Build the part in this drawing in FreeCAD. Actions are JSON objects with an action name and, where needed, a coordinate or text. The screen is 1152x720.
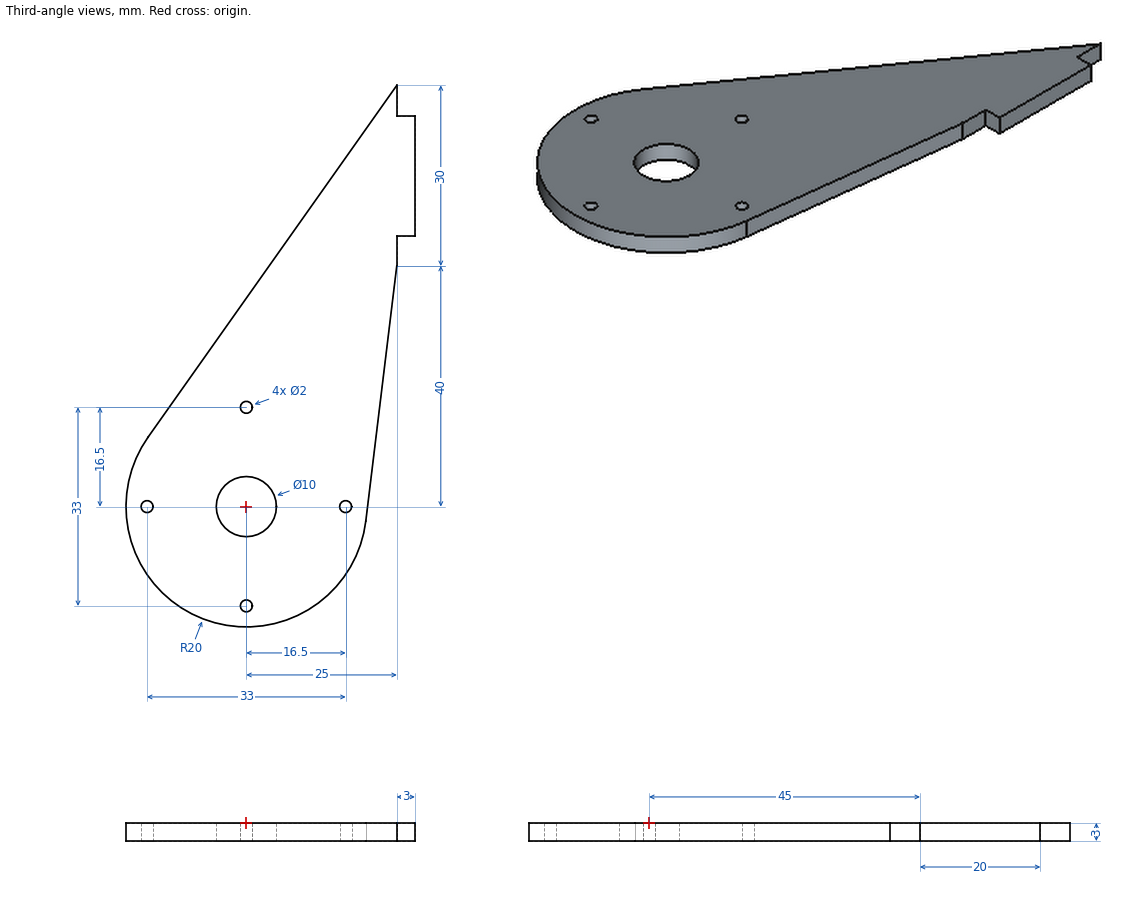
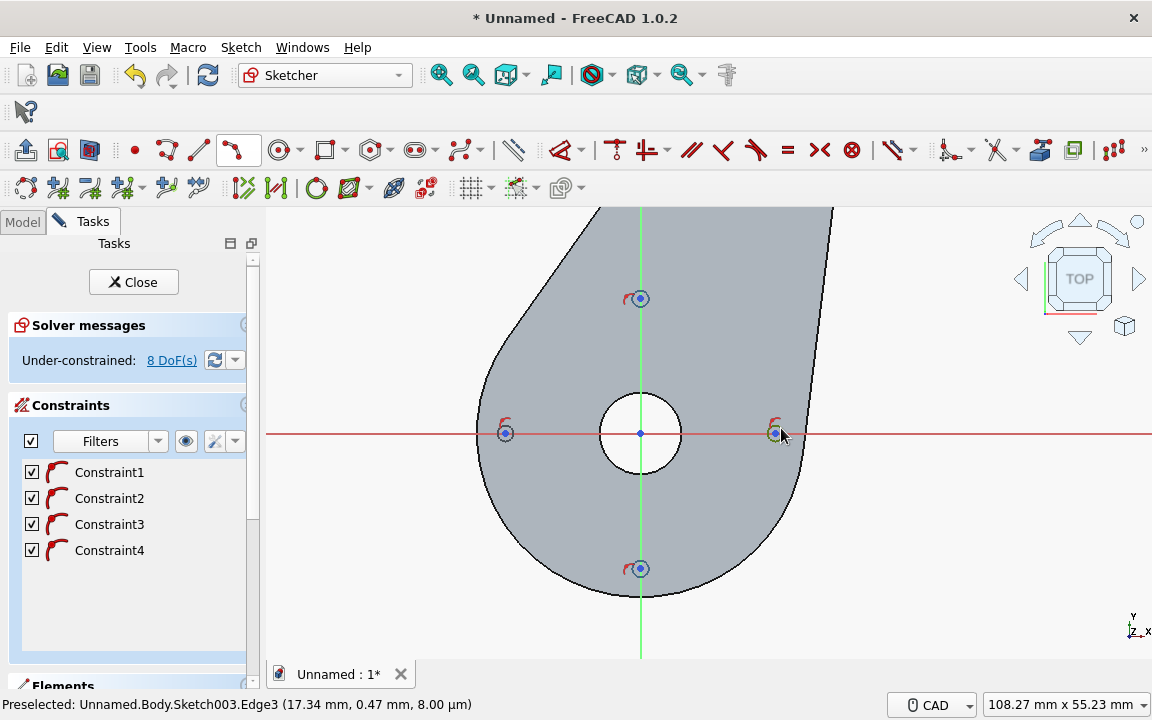
{"action": "scroll", "coordinate": [511, 428], "scroll_direction": "up", "scroll_amount": 5}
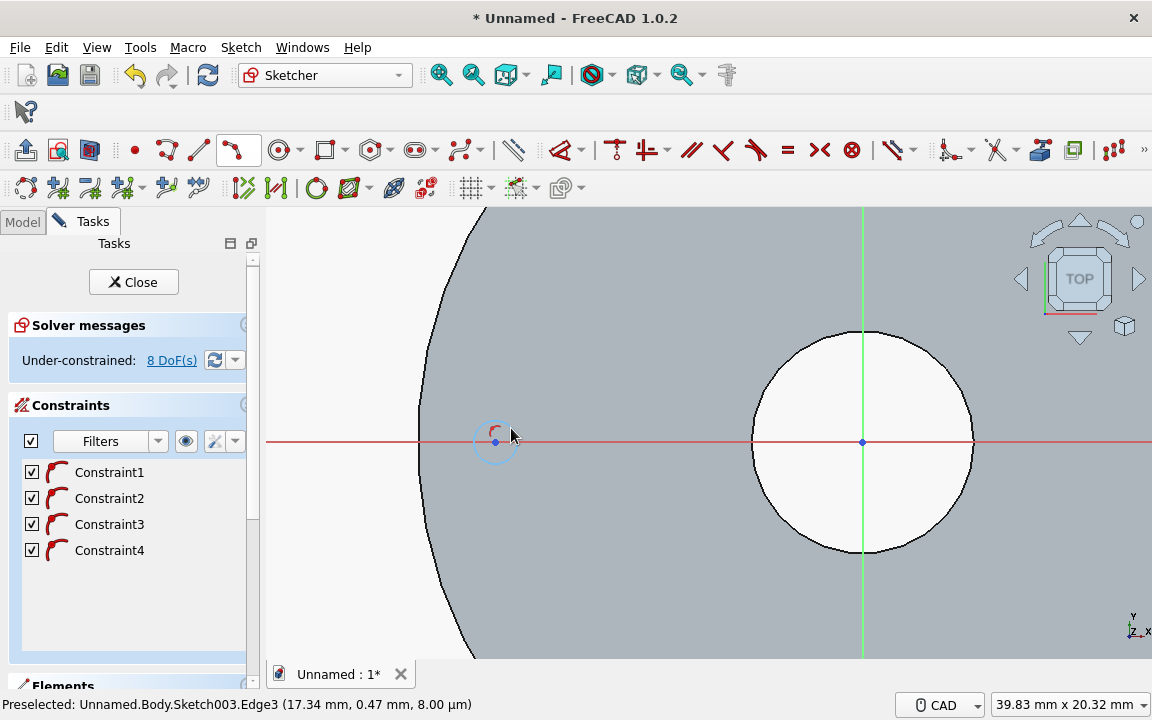
{"action": "left_click", "coordinate": [511, 427]}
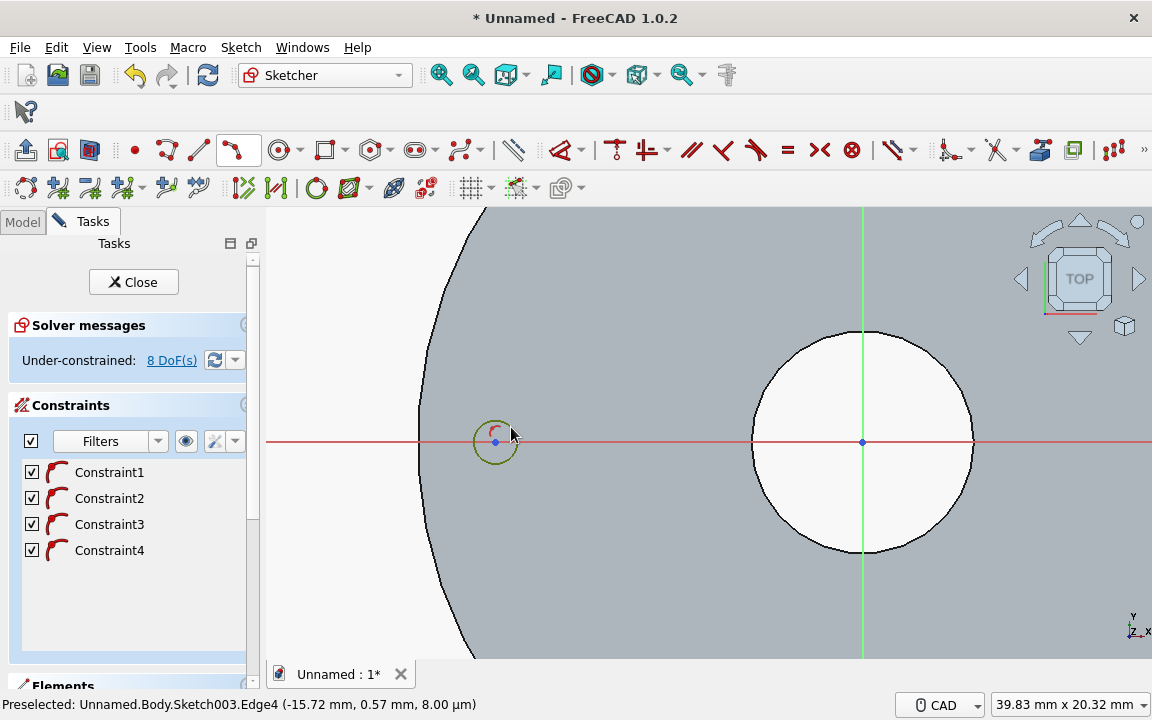
{"action": "left_click", "coordinate": [788, 150]}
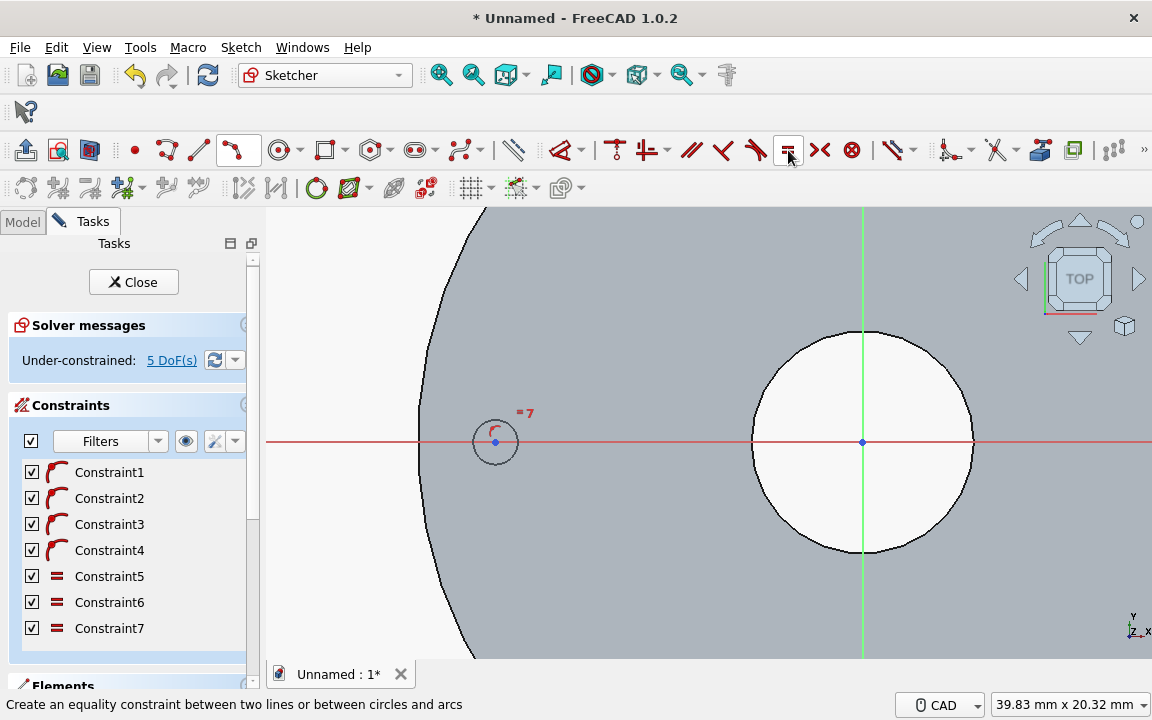
{"action": "left_click", "coordinate": [560, 150]}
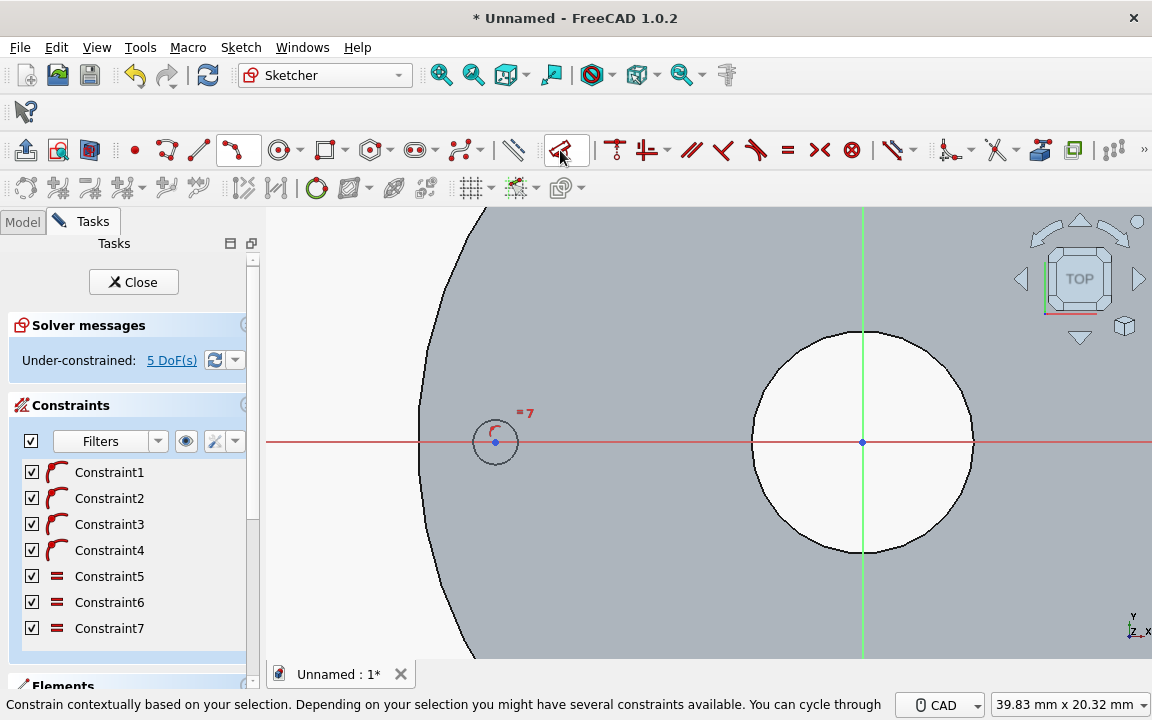
{"action": "scroll", "coordinate": [511, 428], "scroll_direction": "down", "scroll_amount": 5}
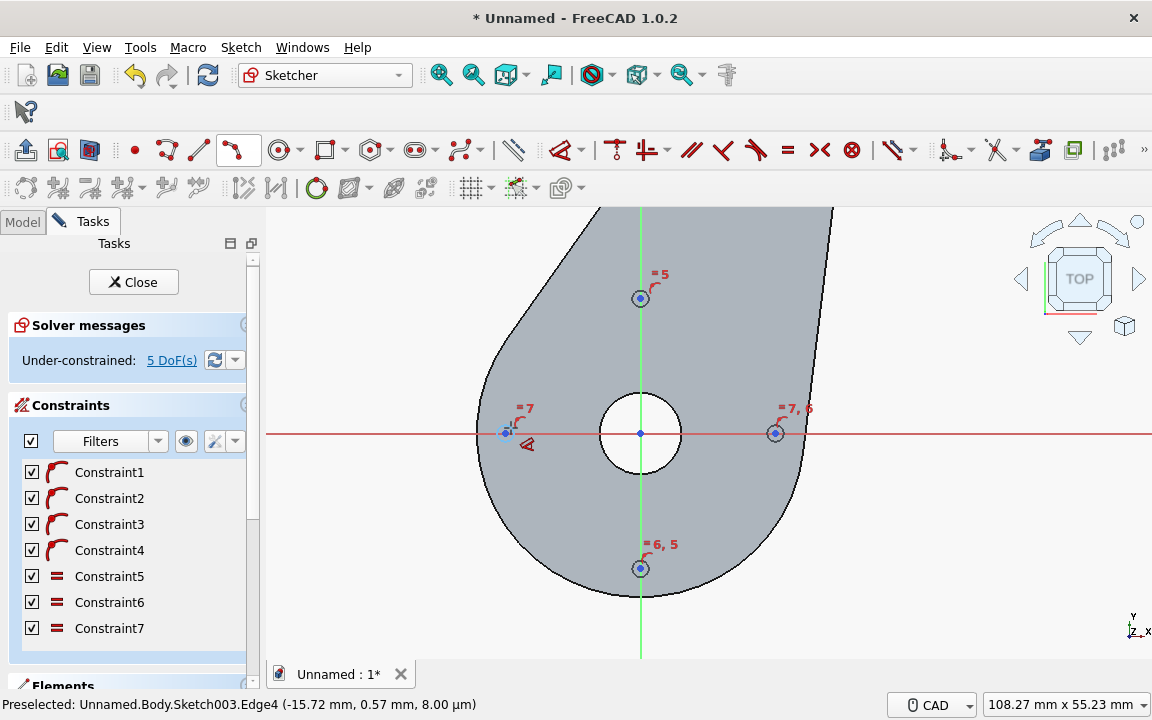
{"action": "scroll", "coordinate": [646, 293], "scroll_direction": "up", "scroll_amount": 5}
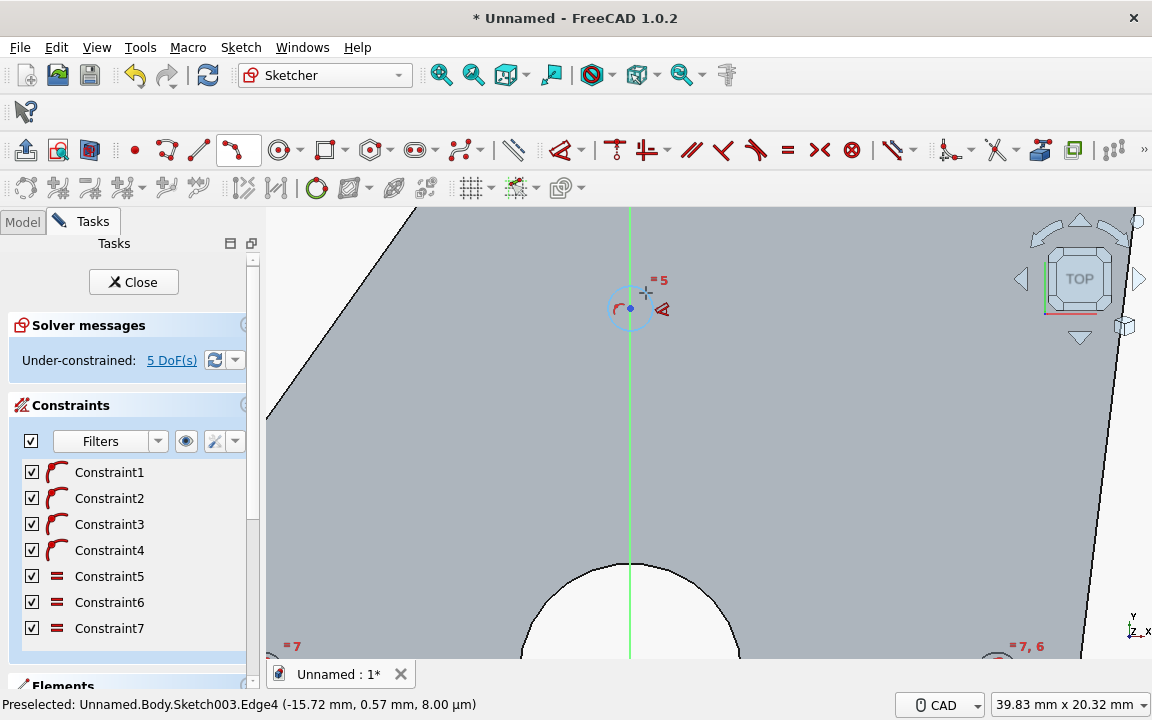
{"action": "left_click", "coordinate": [646, 293]}
{"action": "left_click", "coordinate": [669, 270]}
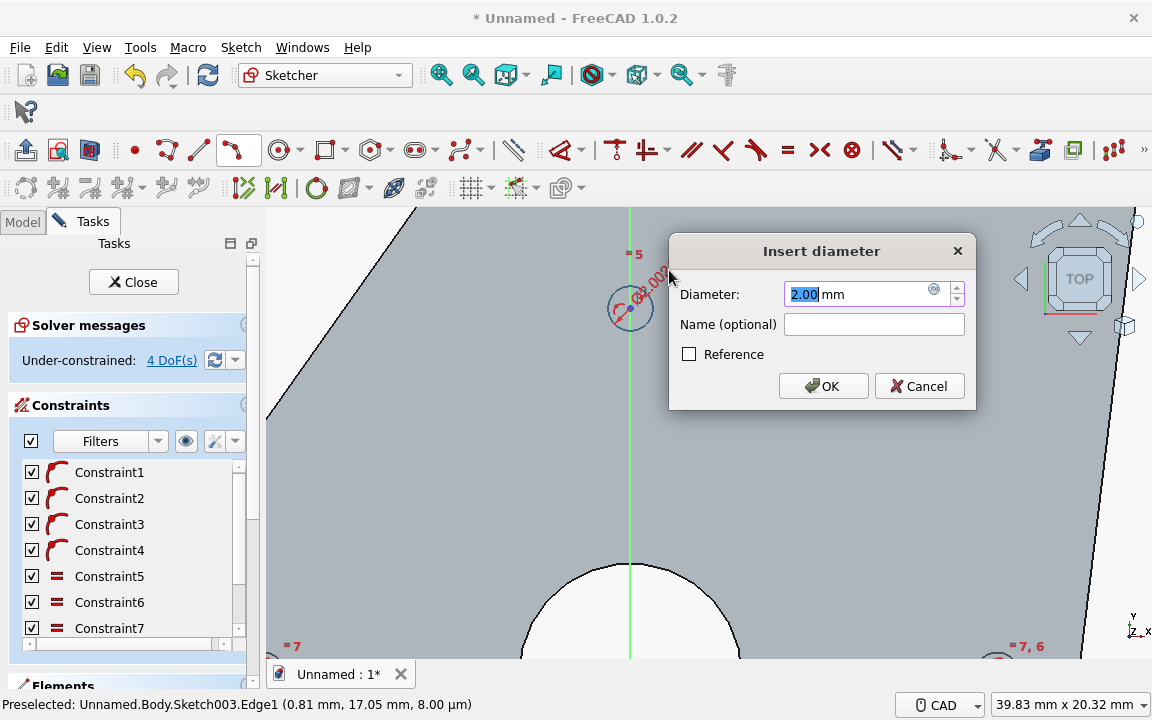
{"action": "type", "text": "2"}
{"action": "key", "text": "Return"}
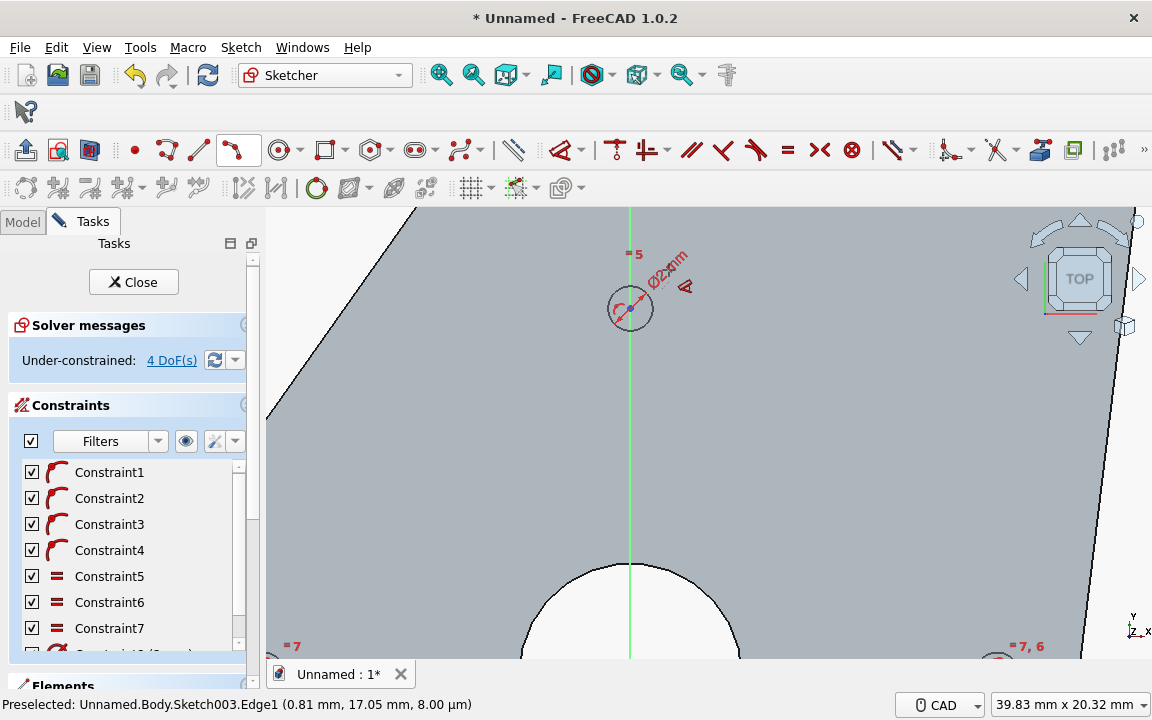
{"action": "left_click", "coordinate": [630, 309]}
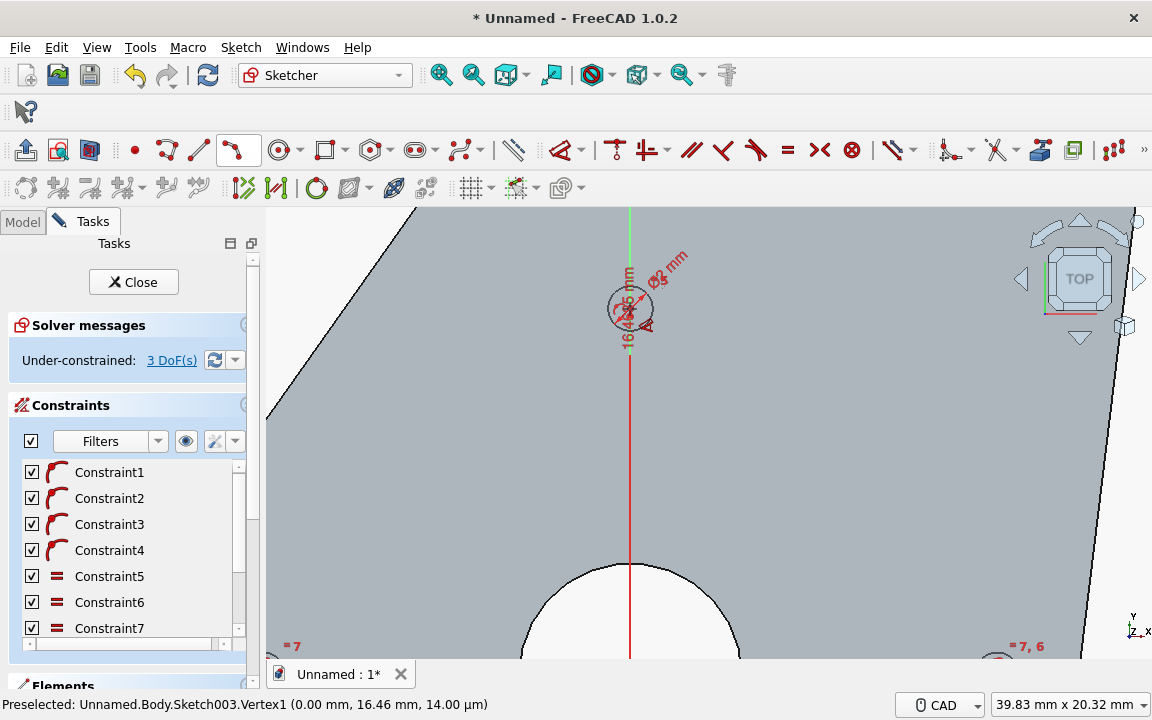
{"action": "scroll", "coordinate": [646, 292], "scroll_direction": "down", "scroll_amount": 5}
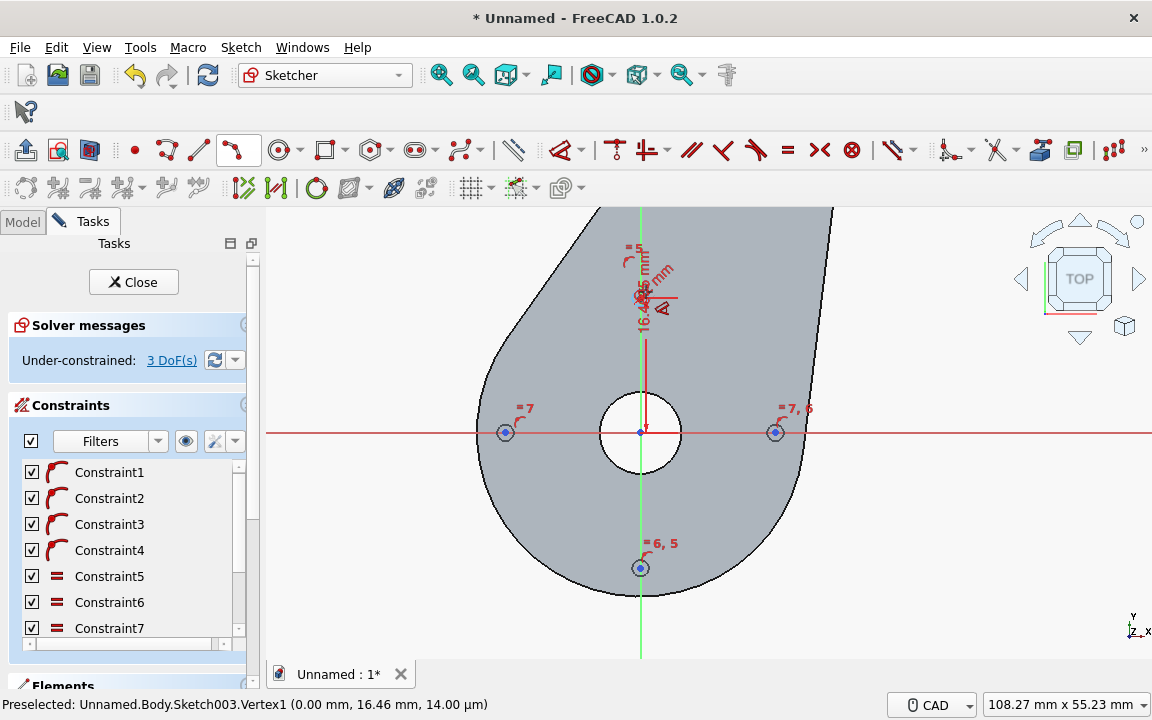
{"action": "left_click", "coordinate": [641, 568]}
{"action": "left_click", "coordinate": [675, 371]}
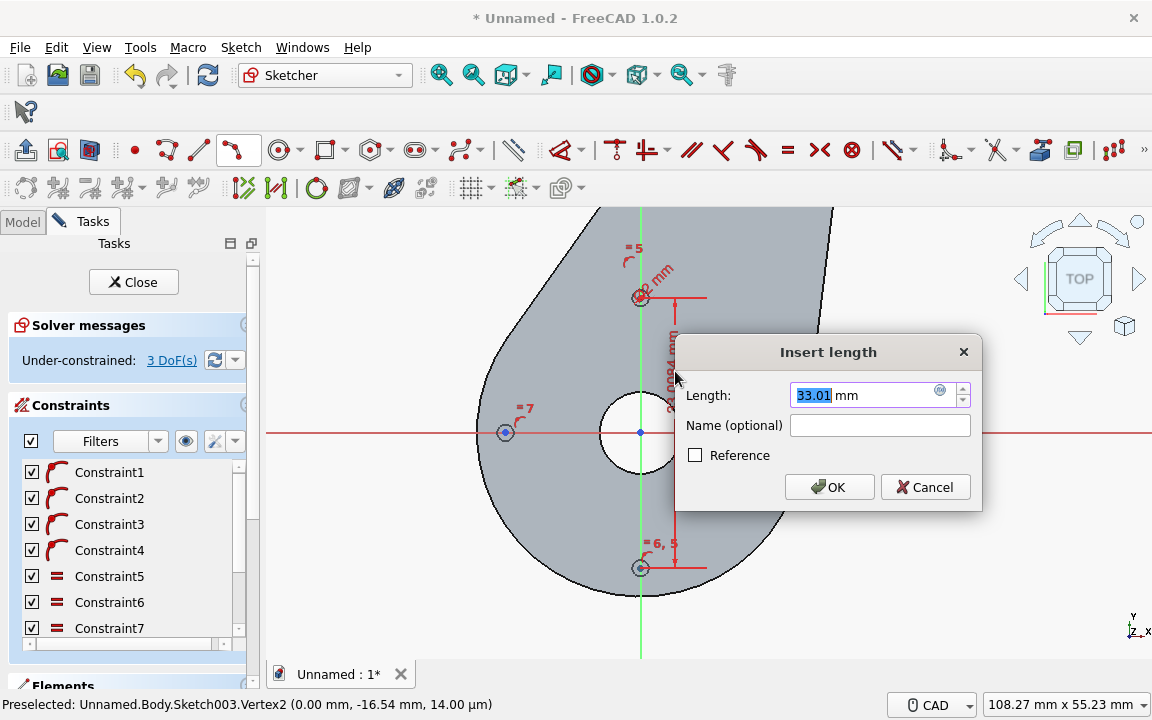
{"action": "type", "text": "33"}
{"action": "key", "text": "Return"}